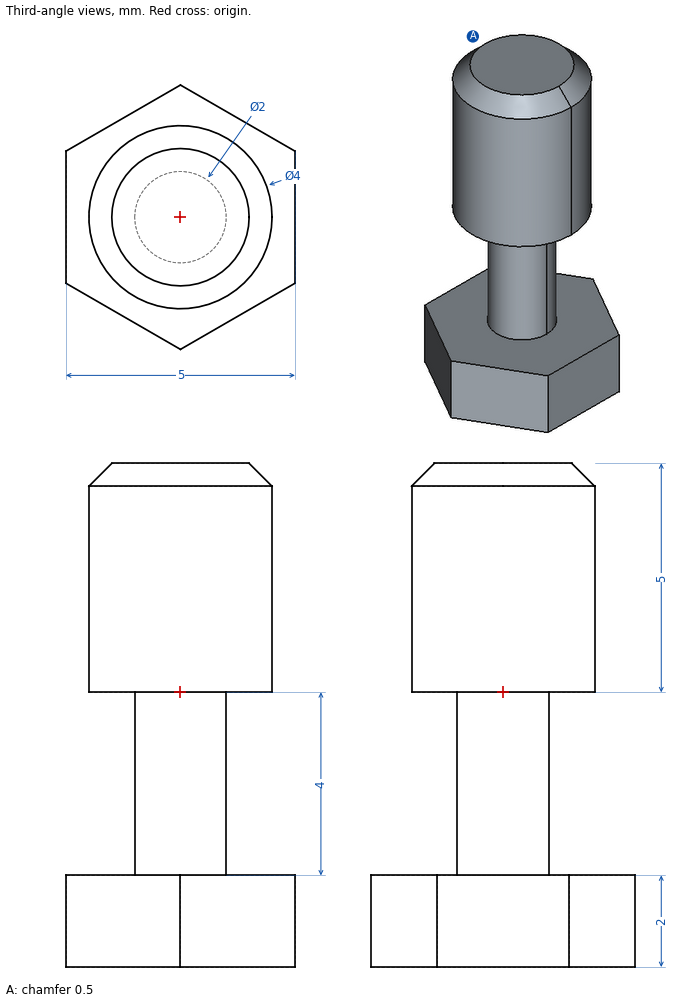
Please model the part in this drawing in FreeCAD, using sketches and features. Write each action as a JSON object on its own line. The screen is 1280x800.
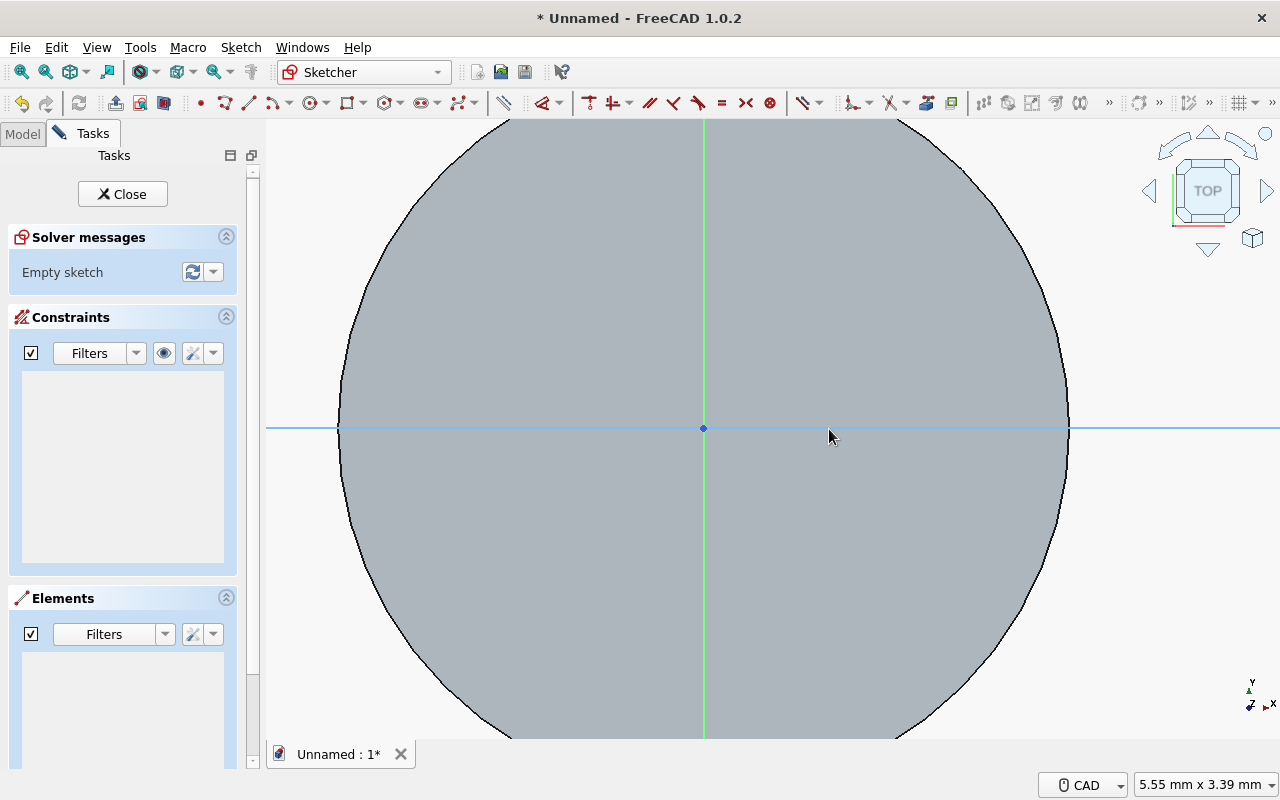
{"action": "left_click", "coordinate": [310, 104]}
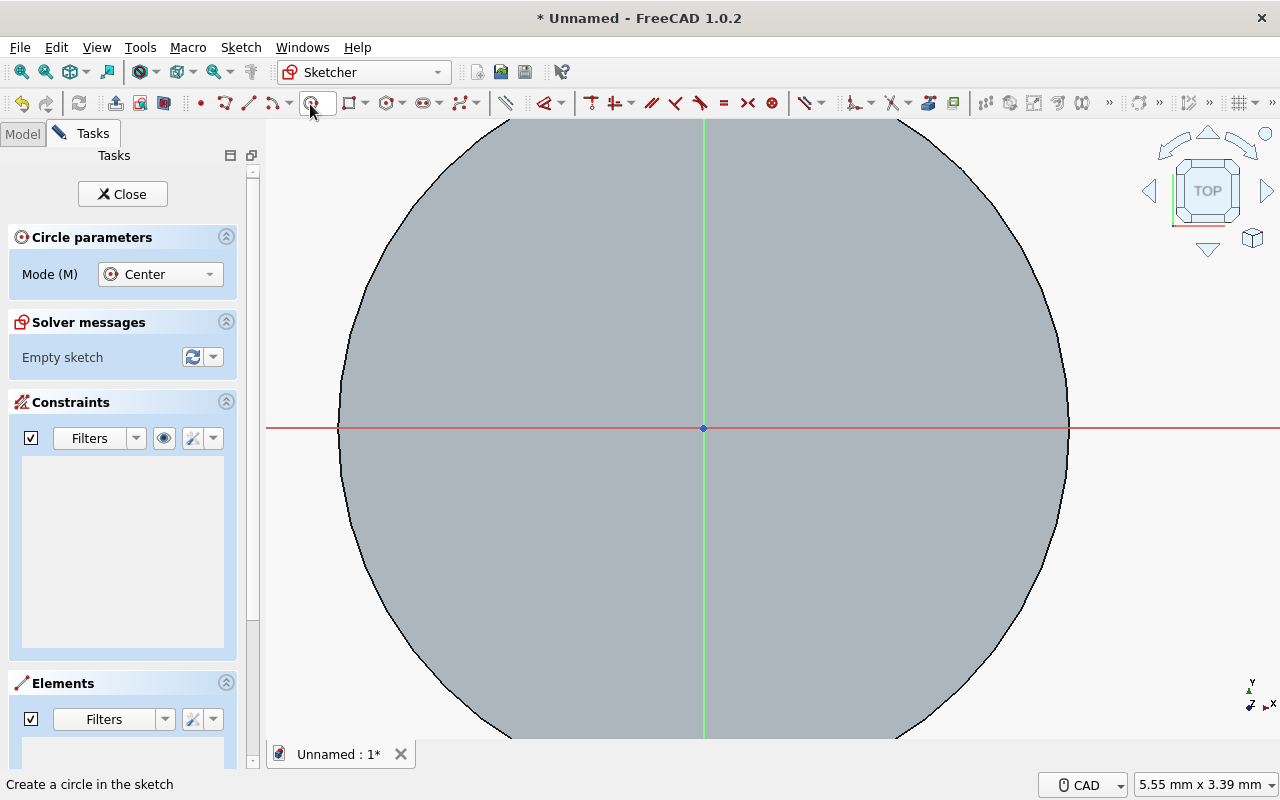
{"action": "left_click", "coordinate": [704, 428]}
{"action": "left_click", "coordinate": [833, 299]}
{"action": "key", "text": "Escape"}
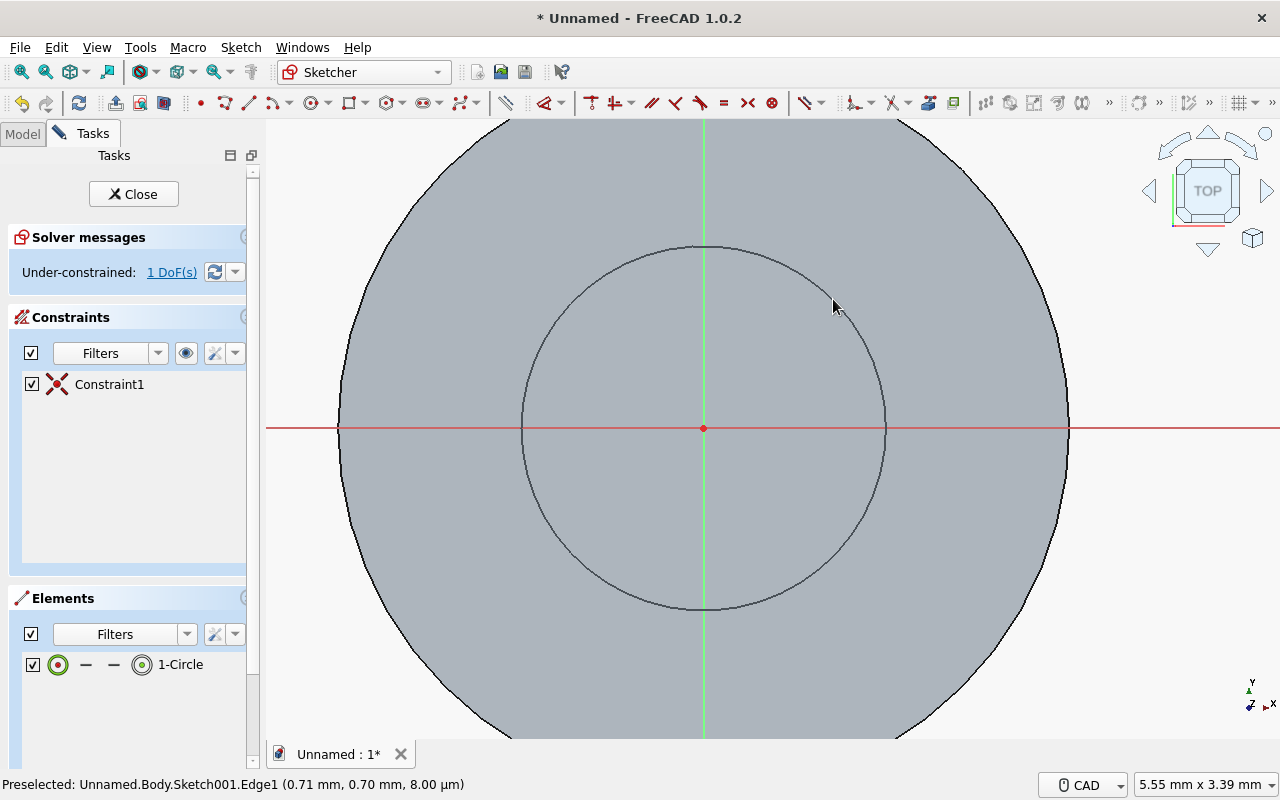
{"action": "left_click", "coordinate": [544, 104]}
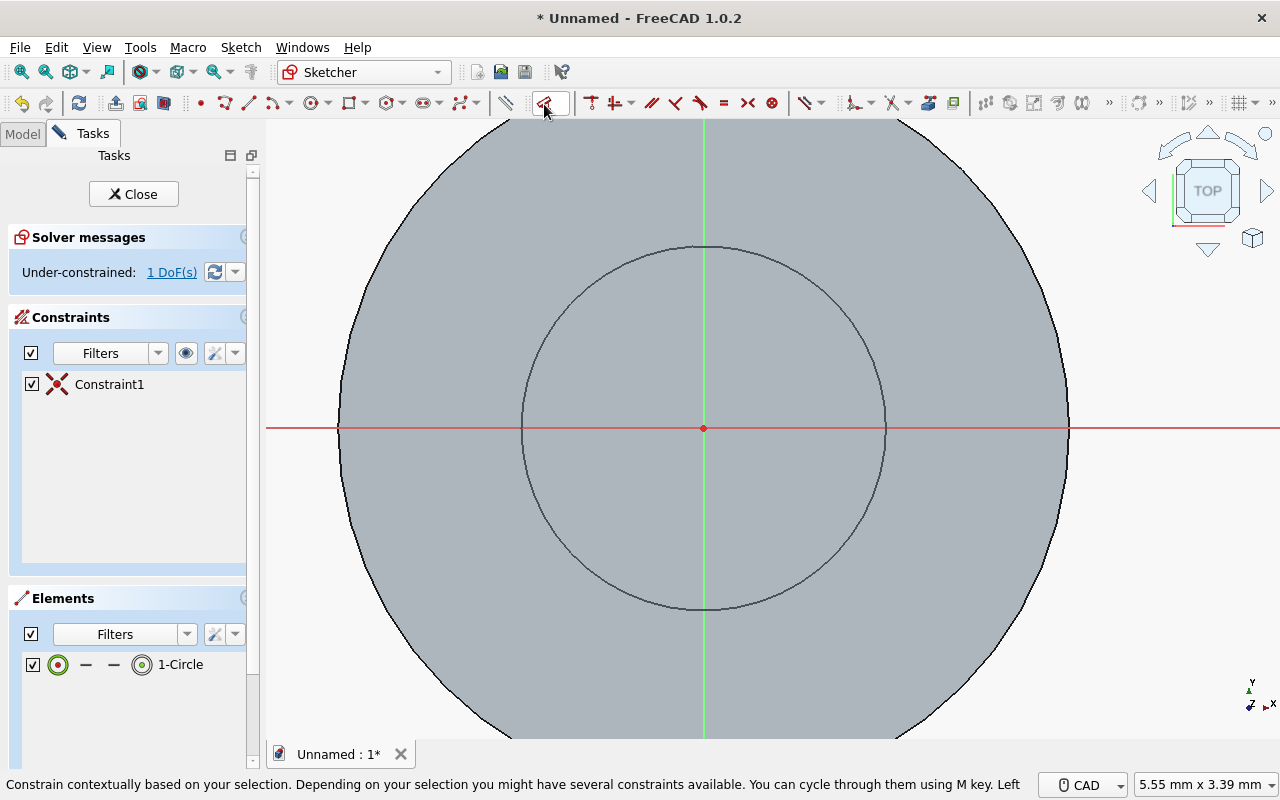
{"action": "left_click", "coordinate": [832, 299]}
{"action": "left_click", "coordinate": [855, 276]}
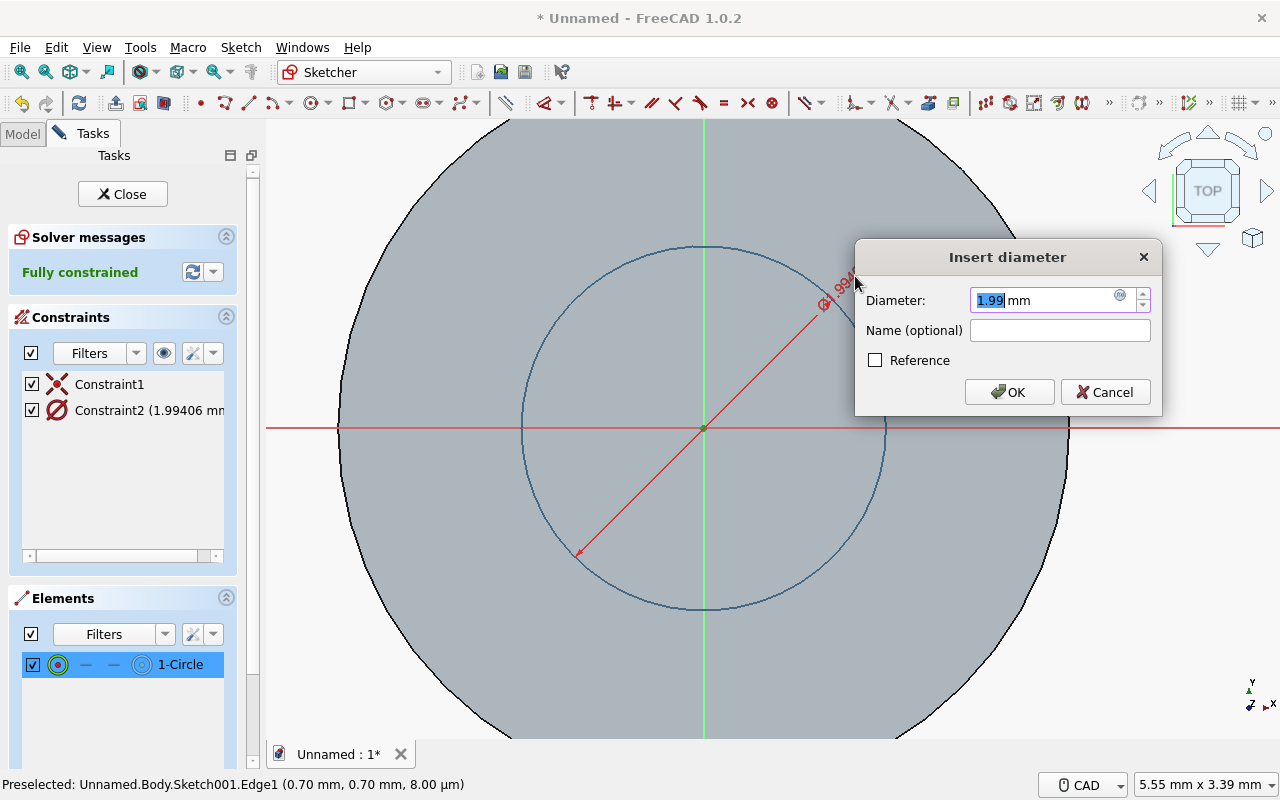
{"action": "type", "text": "2"}
{"action": "key", "text": "Return"}
{"action": "key", "text": "Escape"}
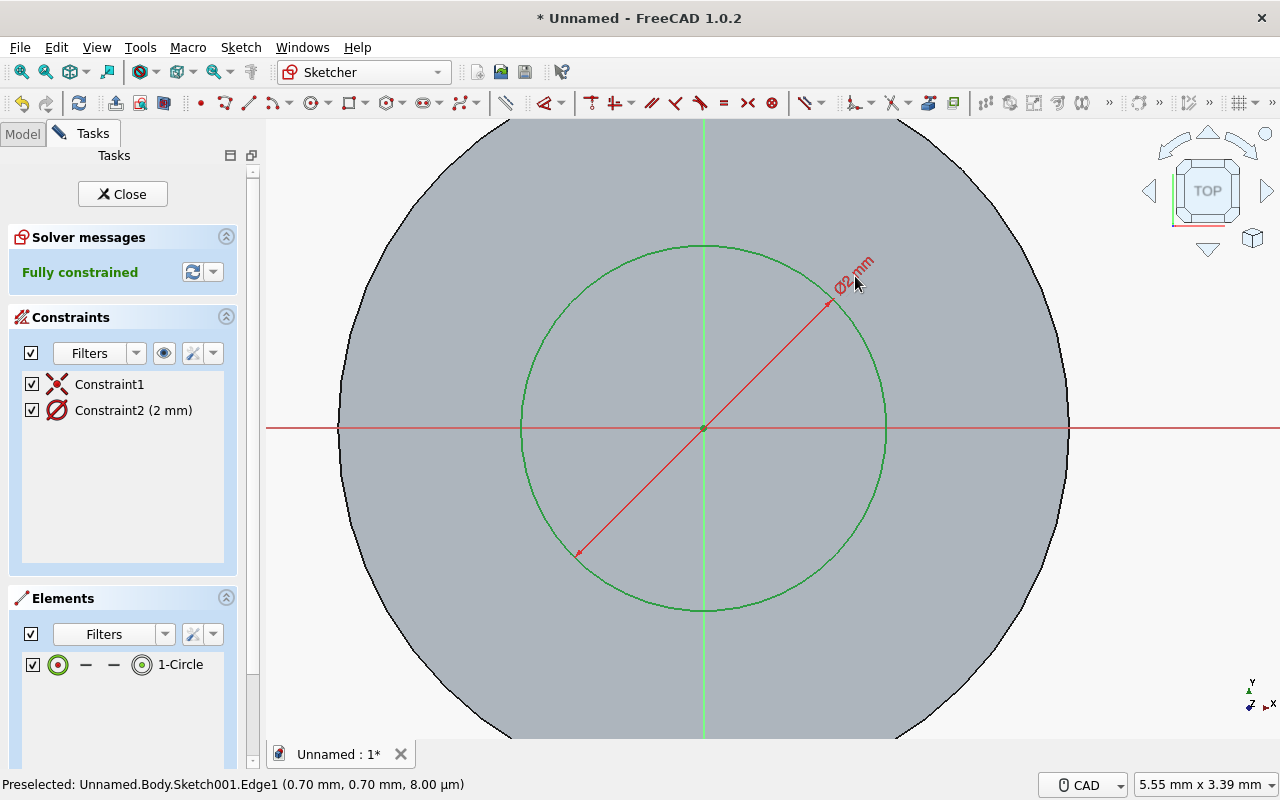
{"action": "left_click", "coordinate": [123, 194]}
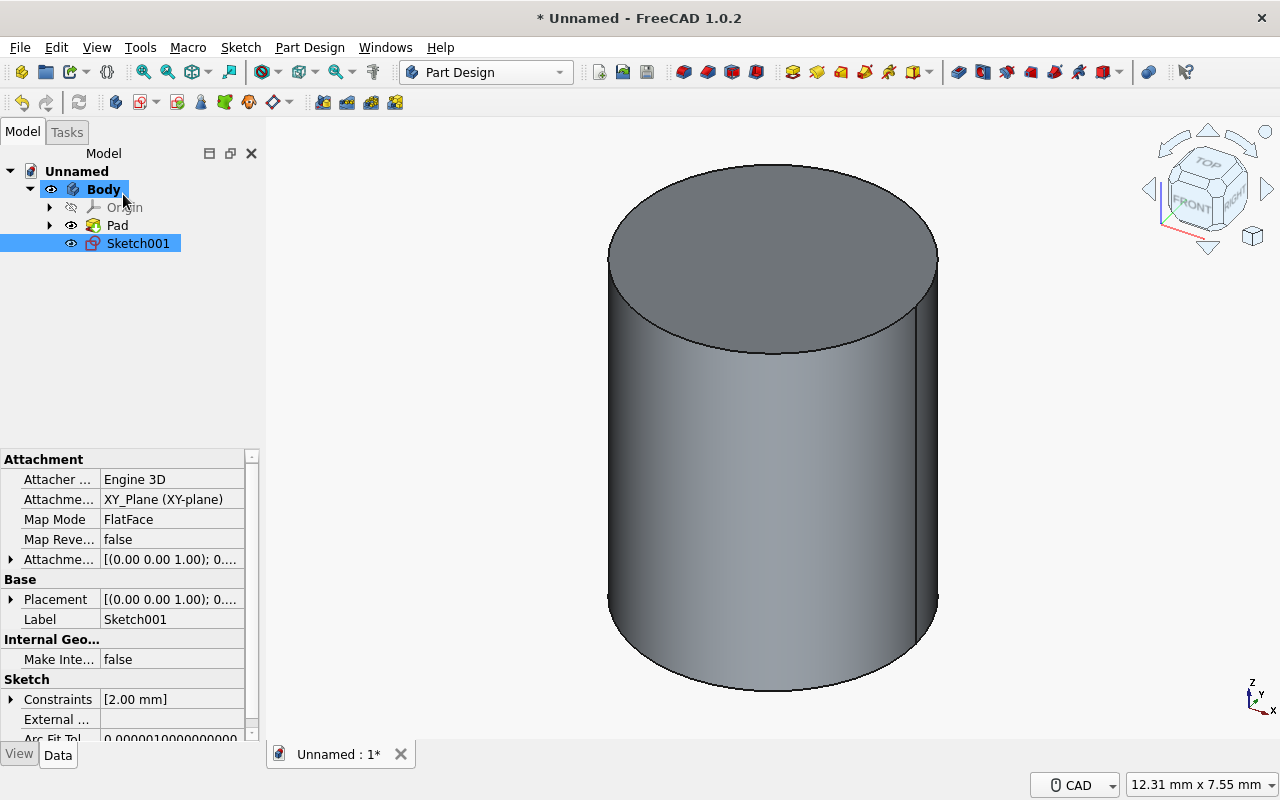
{"action": "left_click", "coordinate": [794, 72]}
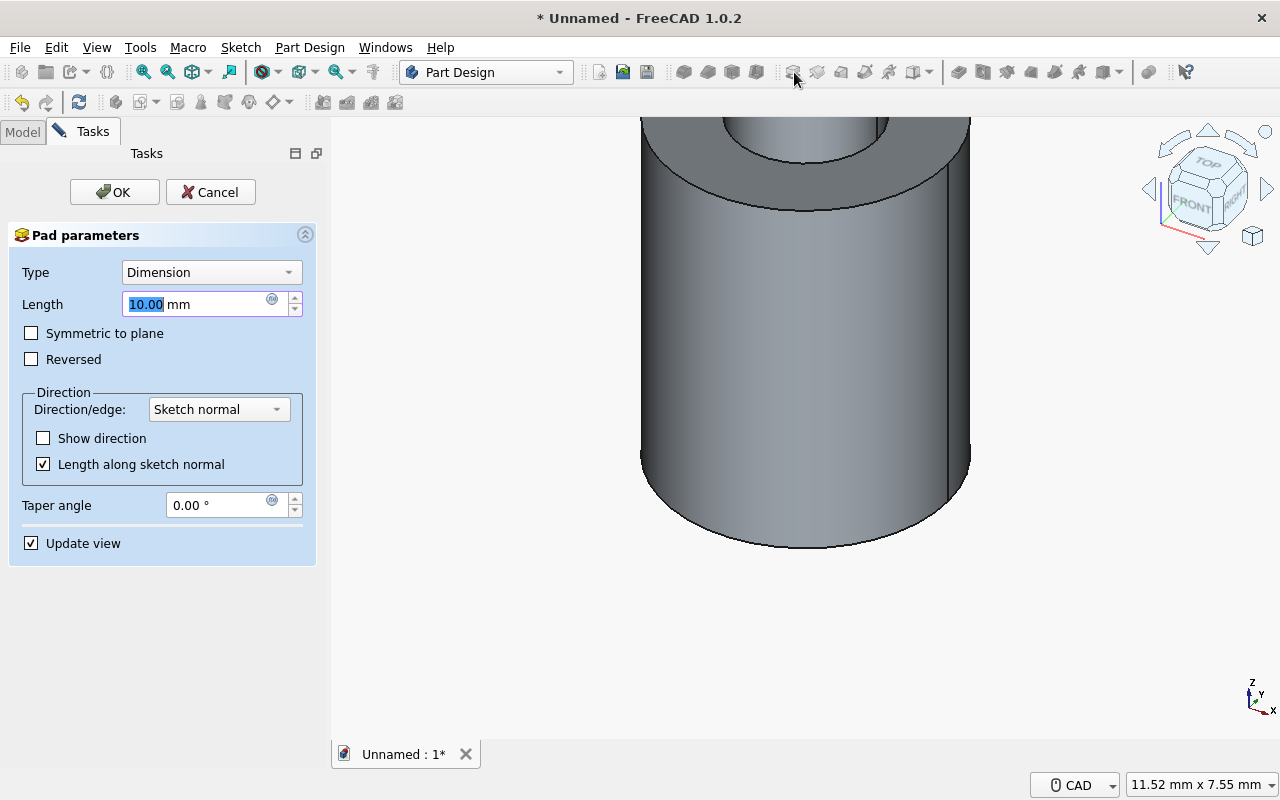
{"action": "type", "text": "4"}
{"action": "key", "text": "Tab"}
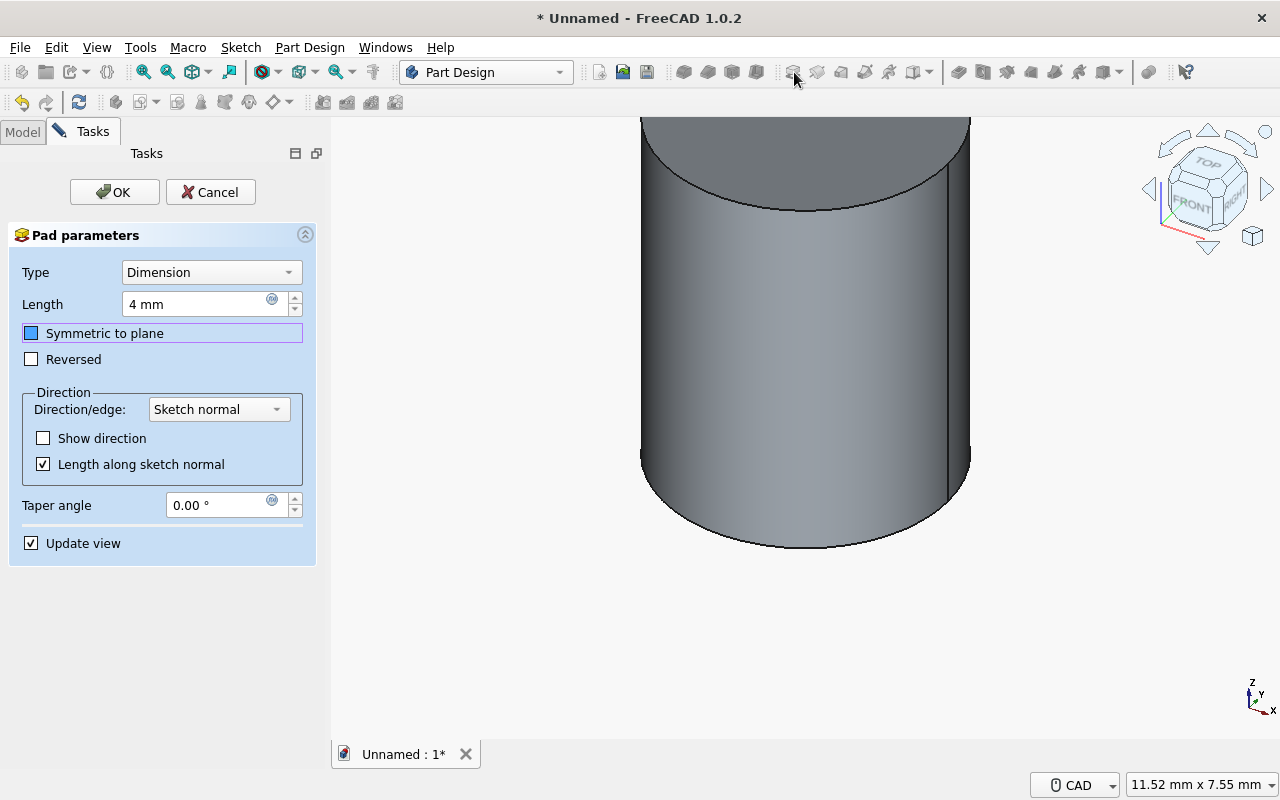
{"action": "left_click", "coordinate": [30, 359]}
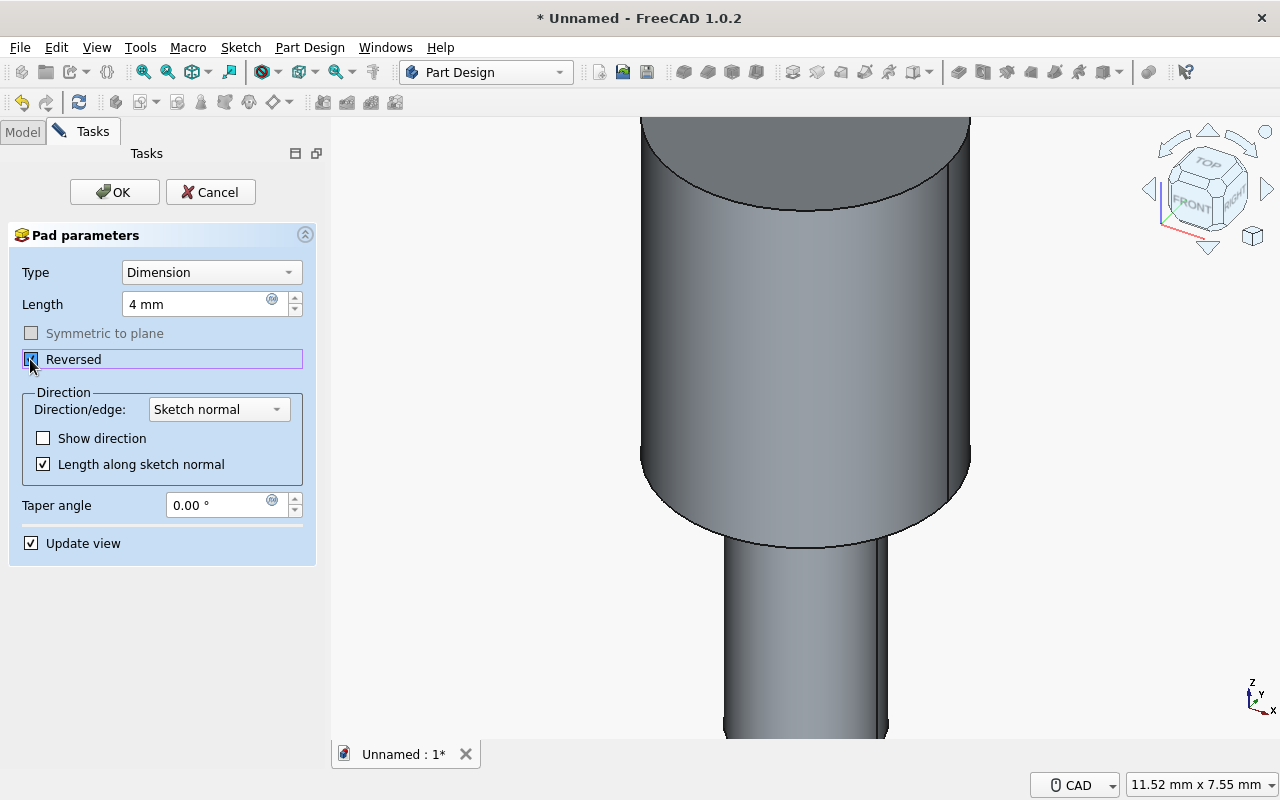
{"action": "left_click", "coordinate": [115, 192]}